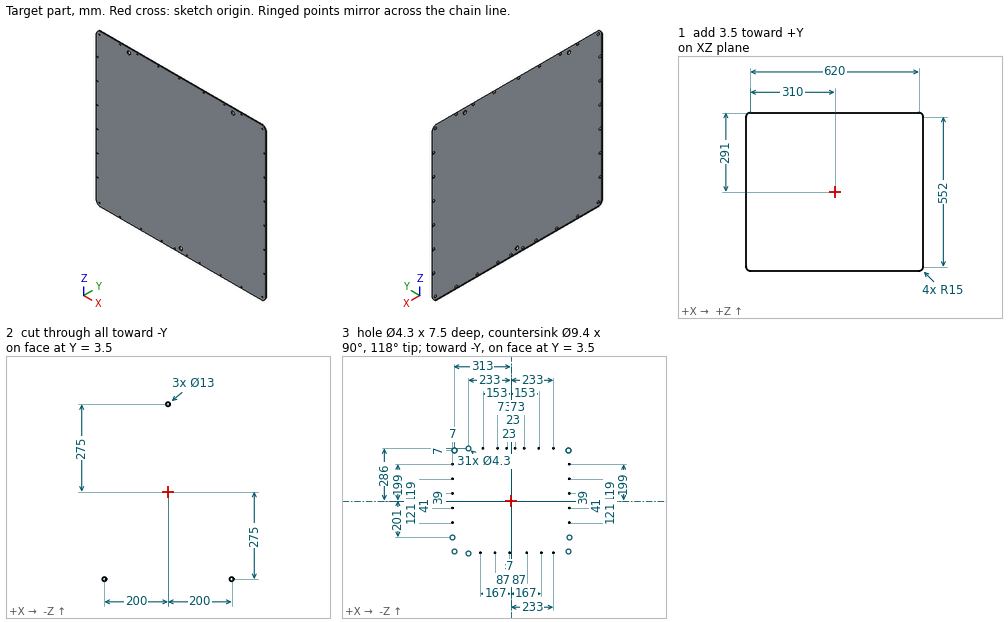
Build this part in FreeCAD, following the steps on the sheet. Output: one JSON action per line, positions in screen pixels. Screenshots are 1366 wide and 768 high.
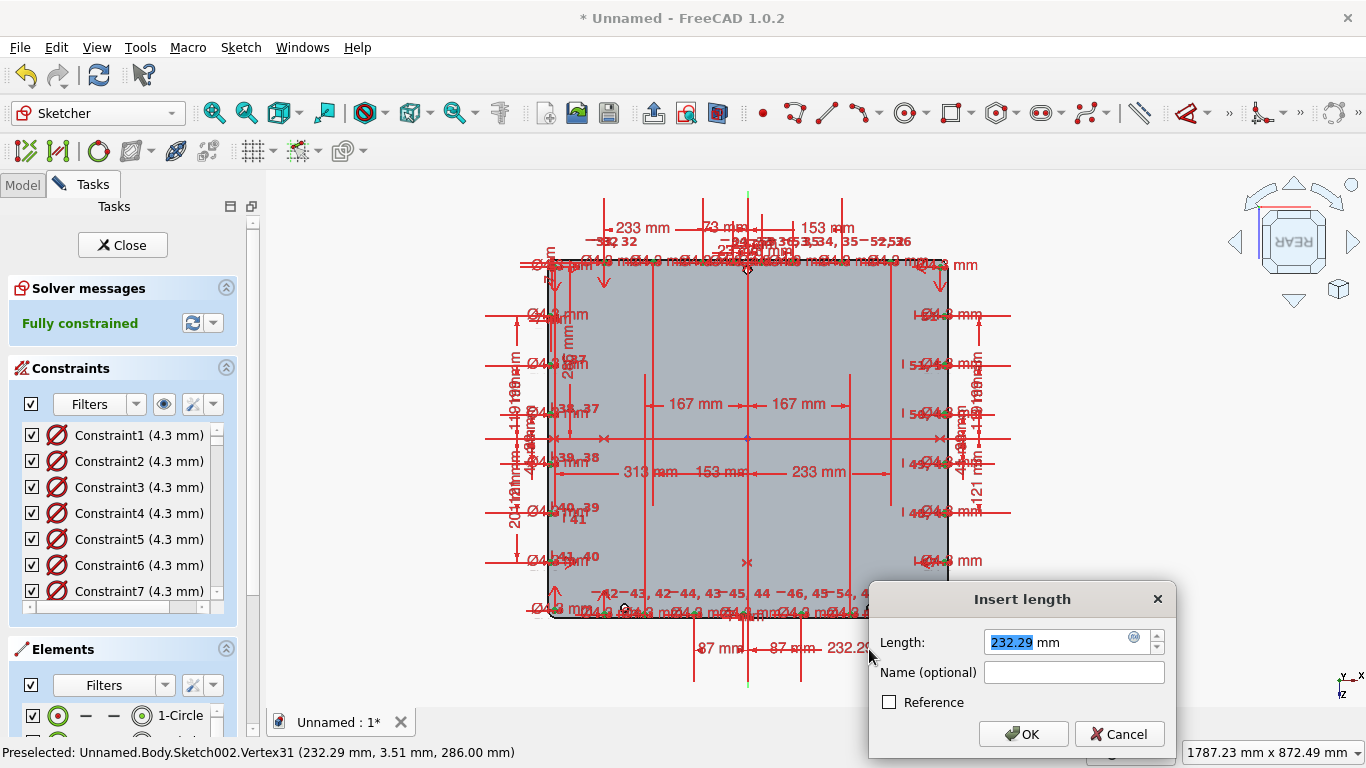
{"action": "type", "text": "233"}
{"action": "key", "text": "Return"}
{"action": "key", "text": "Escape"}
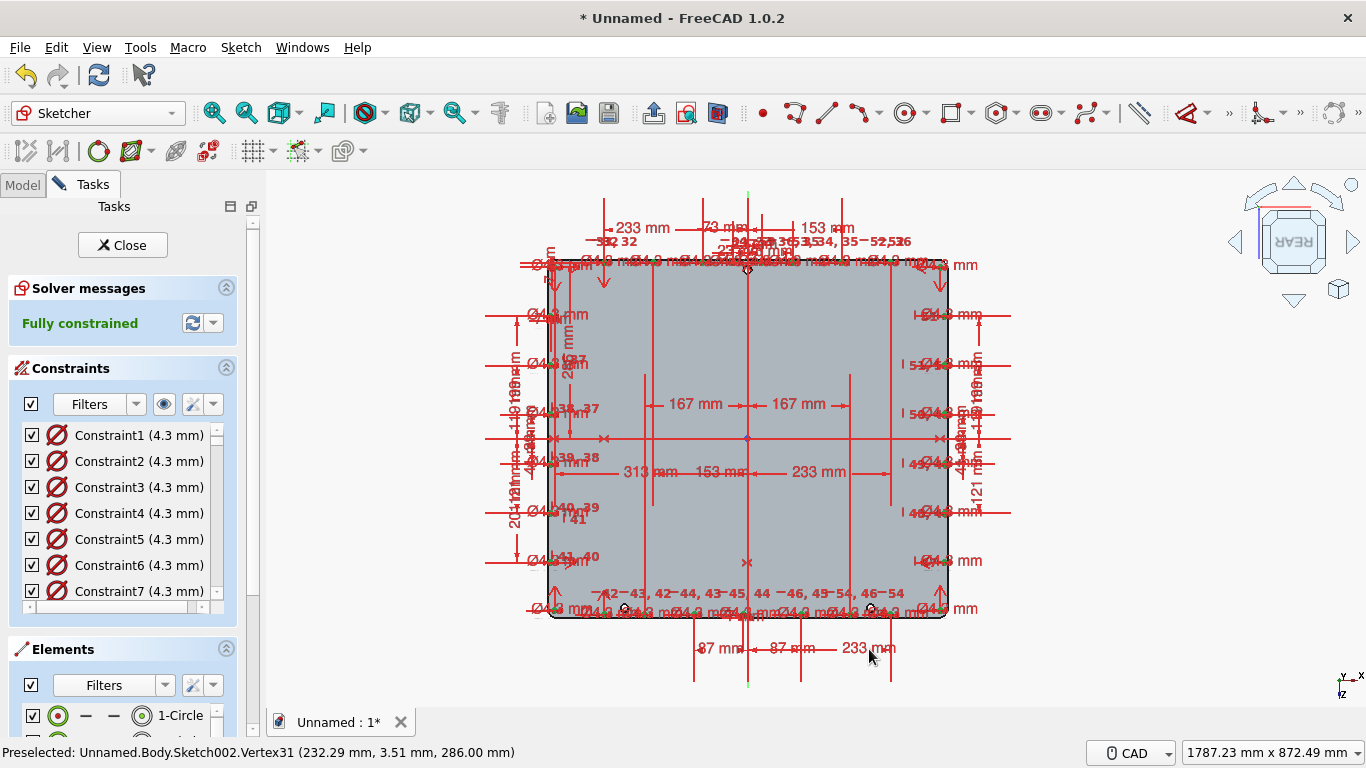
{"action": "left_click", "coordinate": [123, 245]}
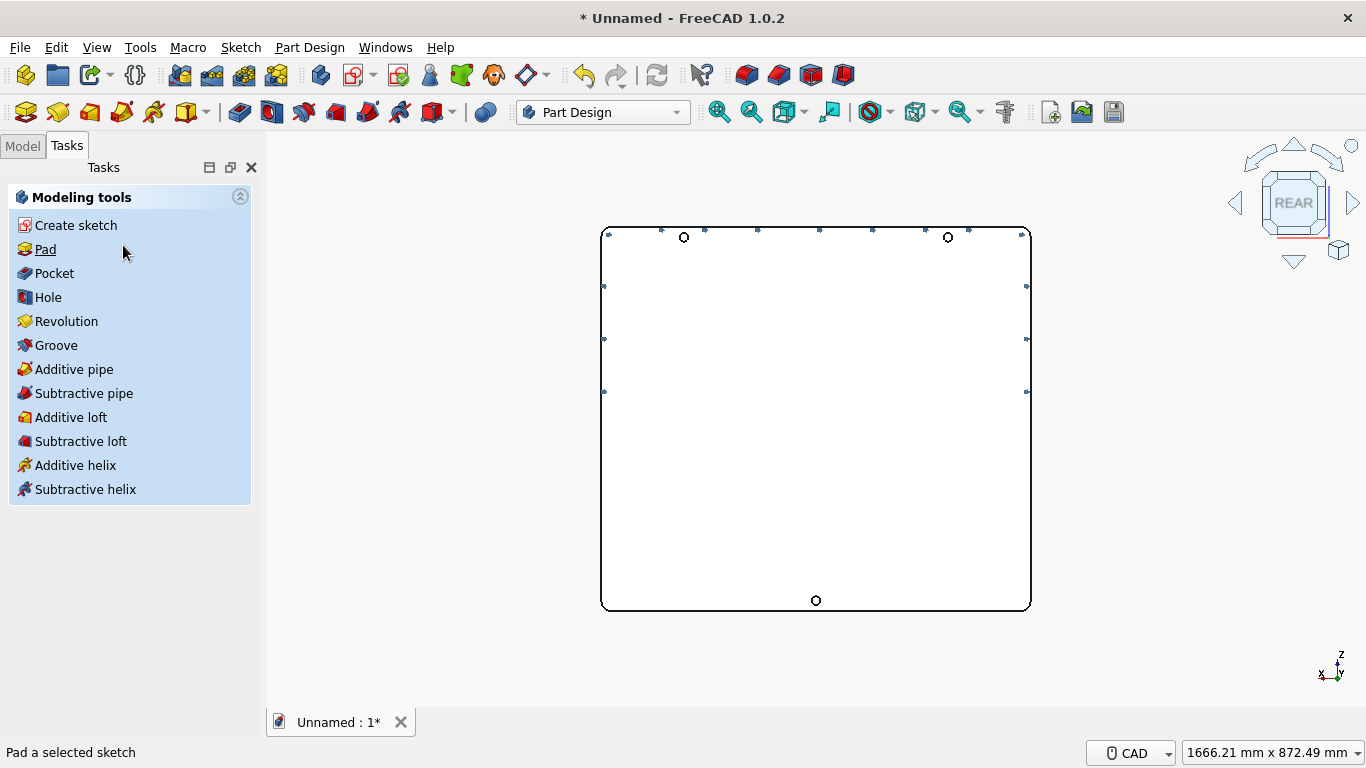
{"action": "left_click", "coordinate": [272, 112]}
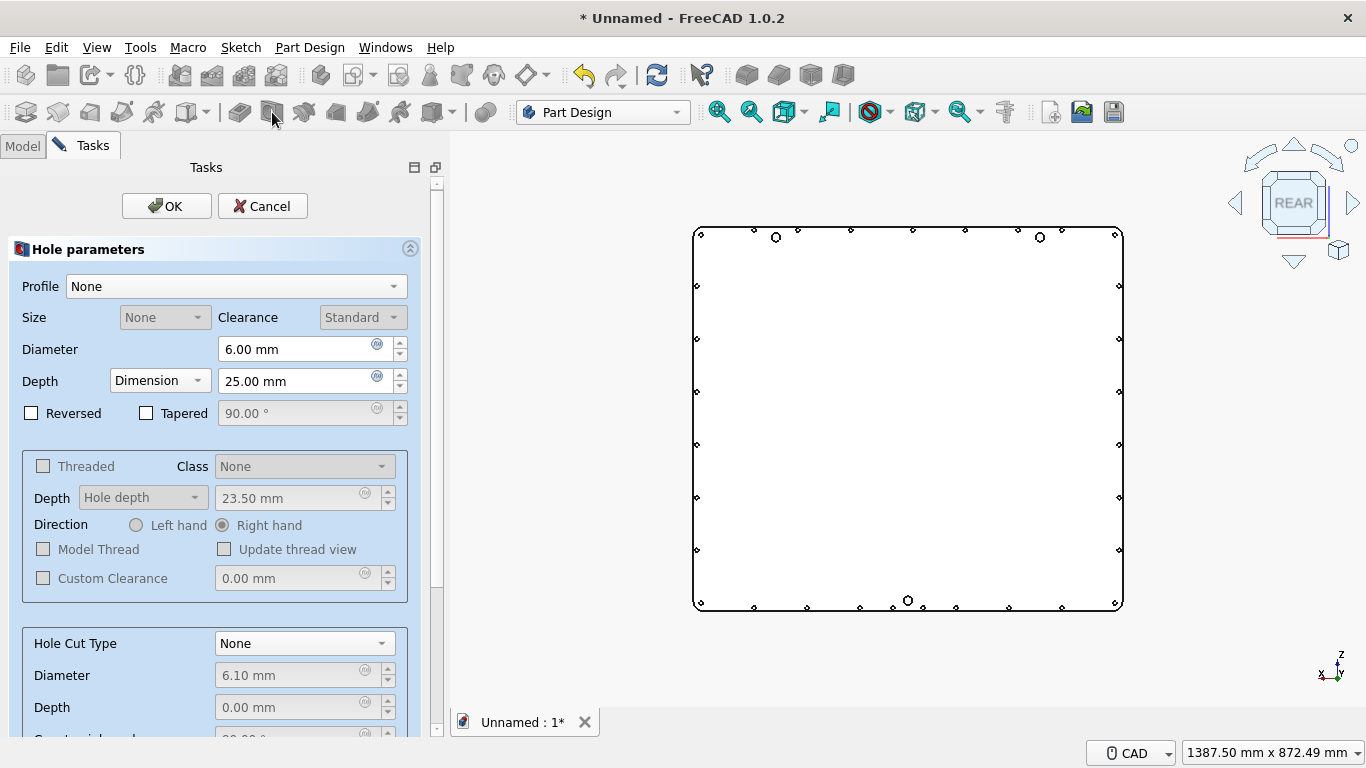
{"action": "triple_click", "coordinate": [305, 349]}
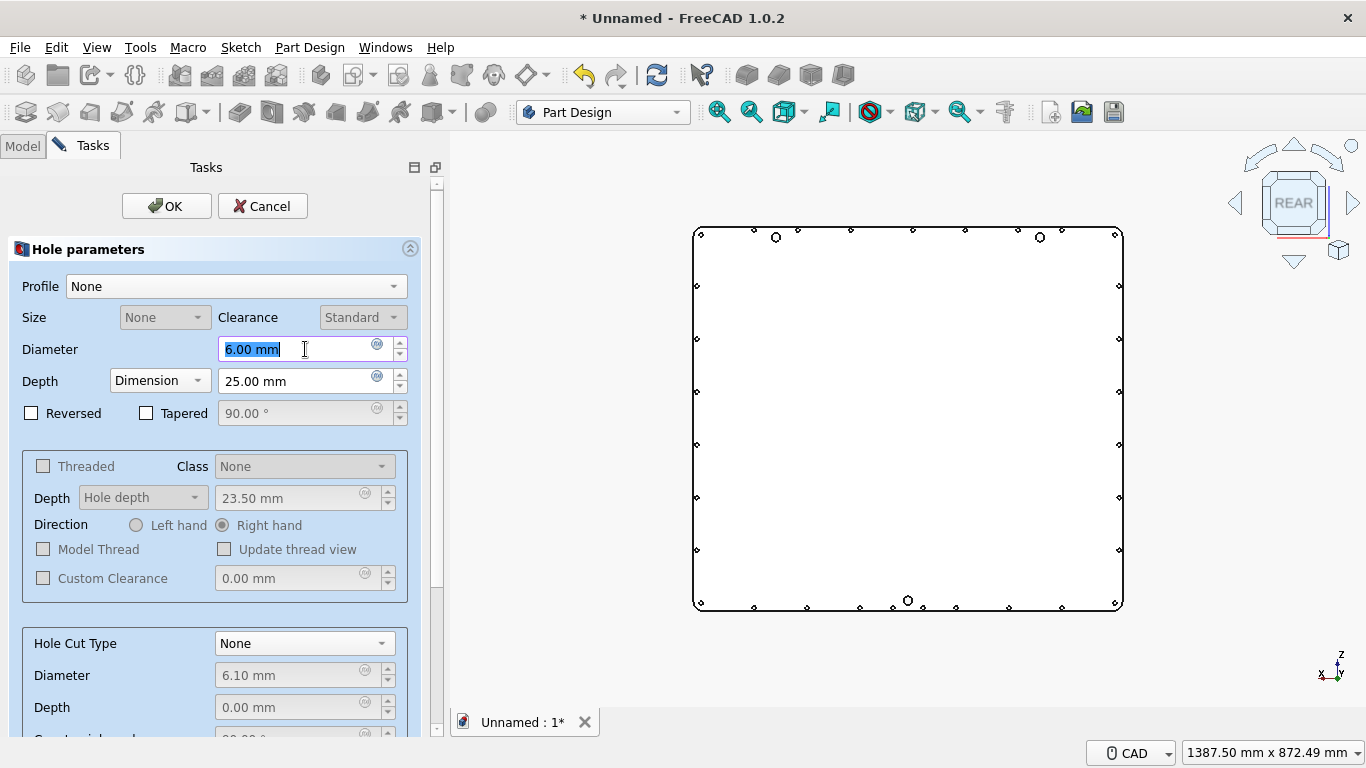
{"action": "type", "text": "4.3"}
{"action": "key", "text": "Tab"}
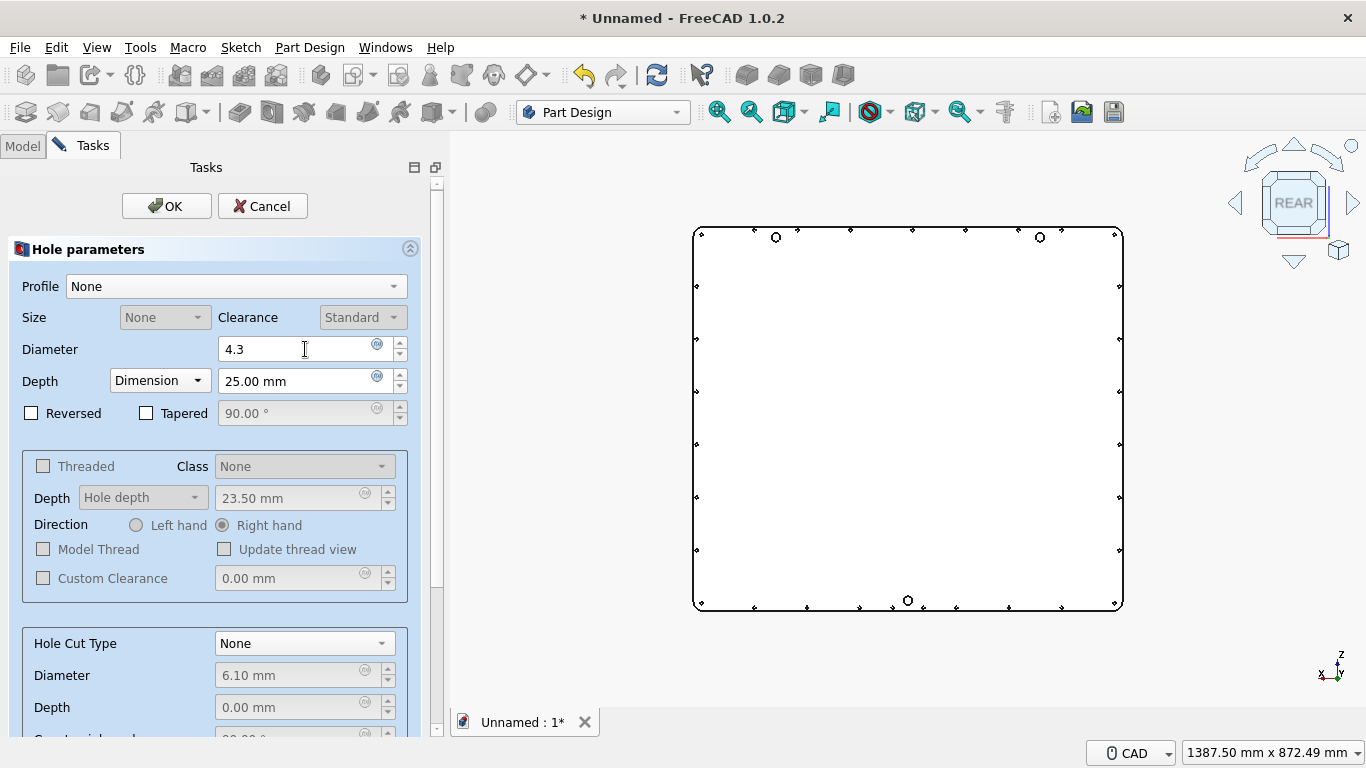
{"action": "triple_click", "coordinate": [305, 381]}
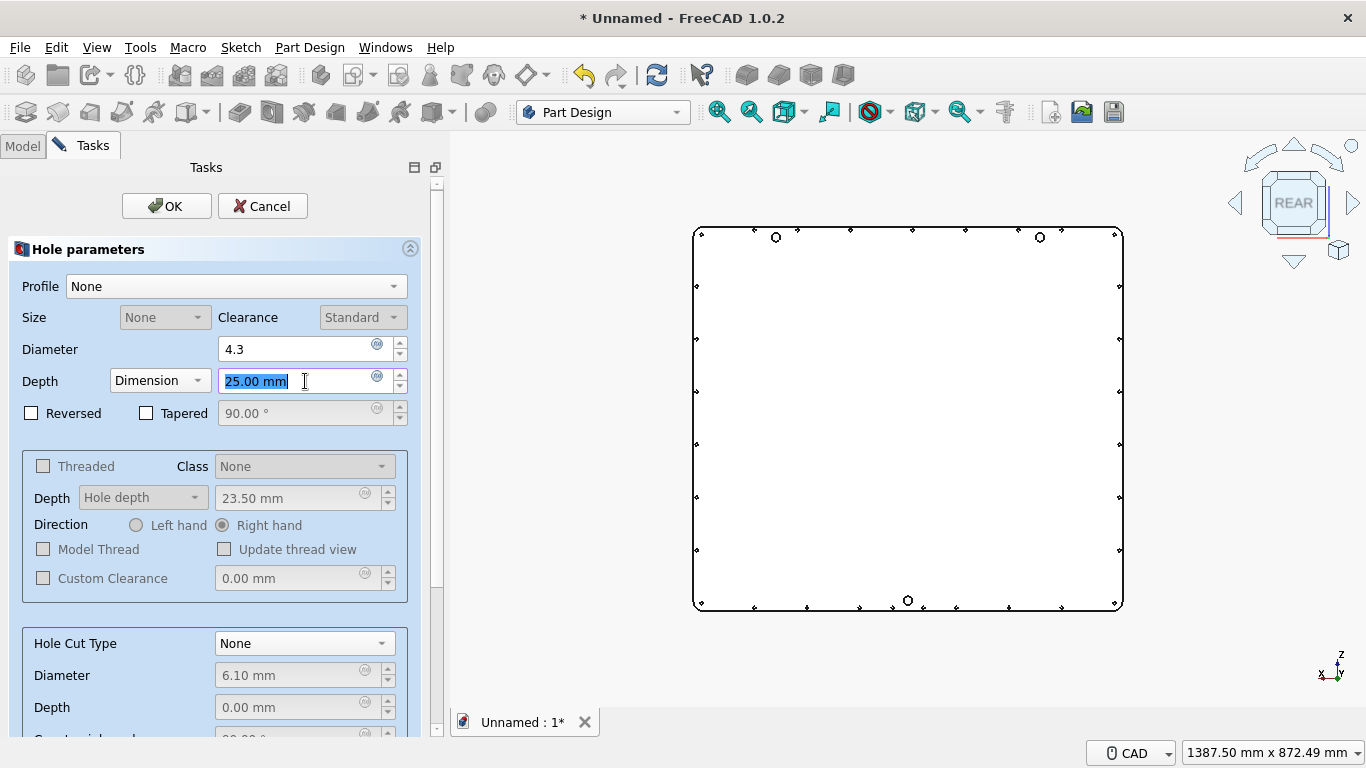
{"action": "type", "text": "7.5"}
{"action": "key", "text": "Tab"}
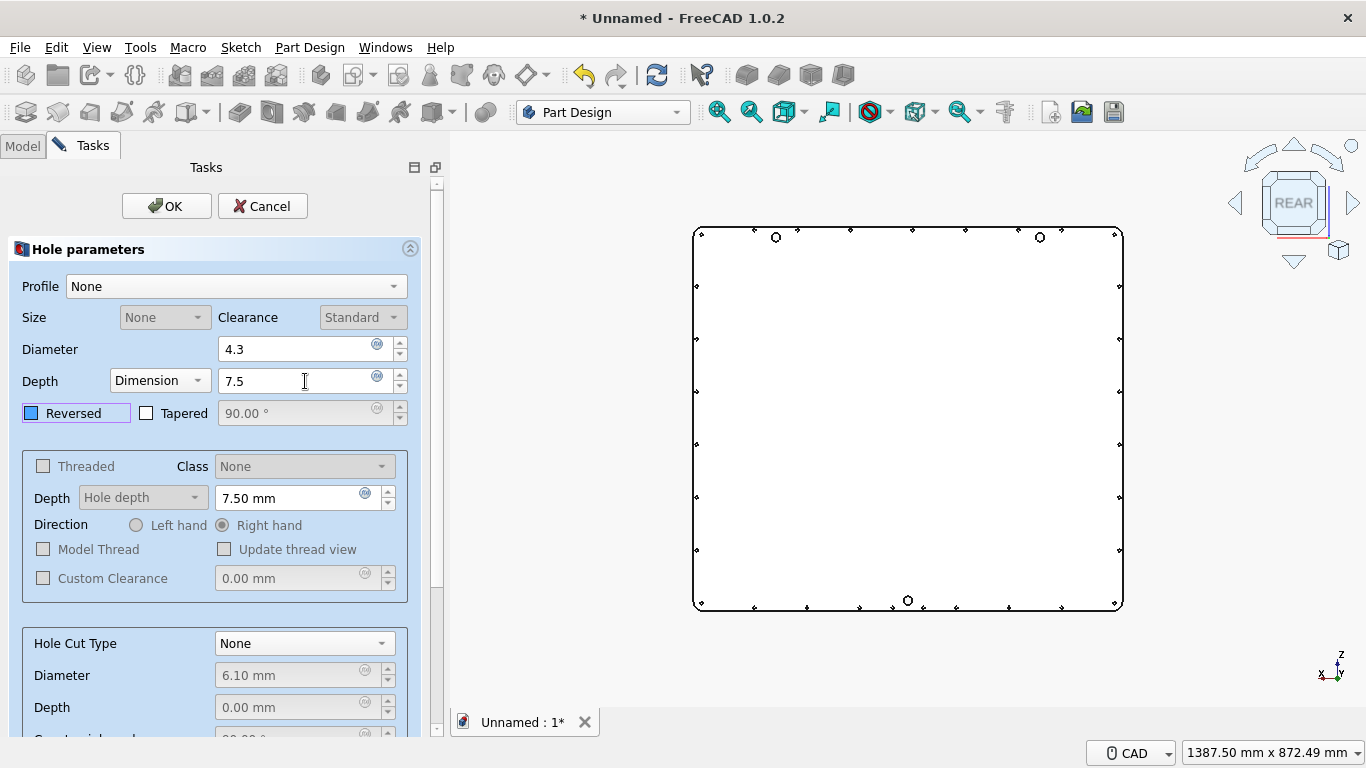
{"action": "left_click", "coordinate": [306, 644]}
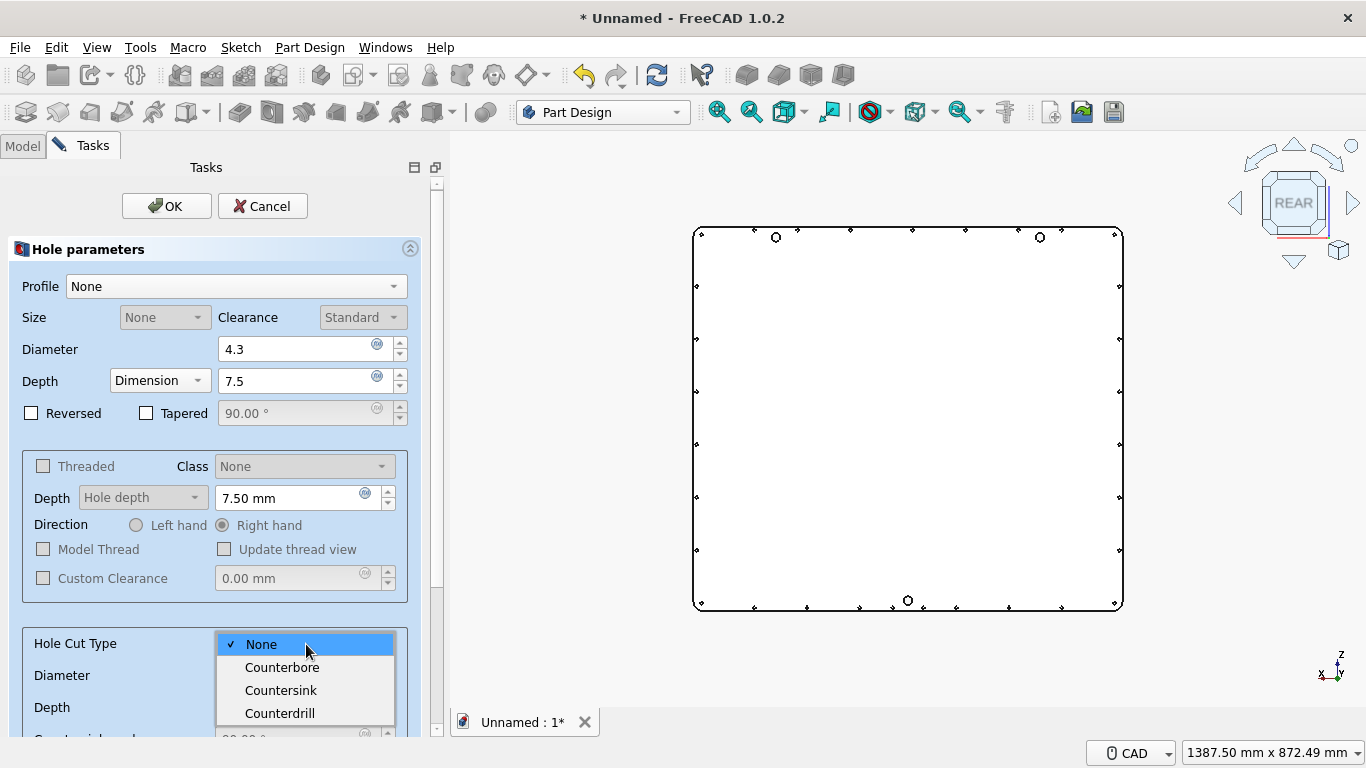
{"action": "left_click", "coordinate": [304, 690]}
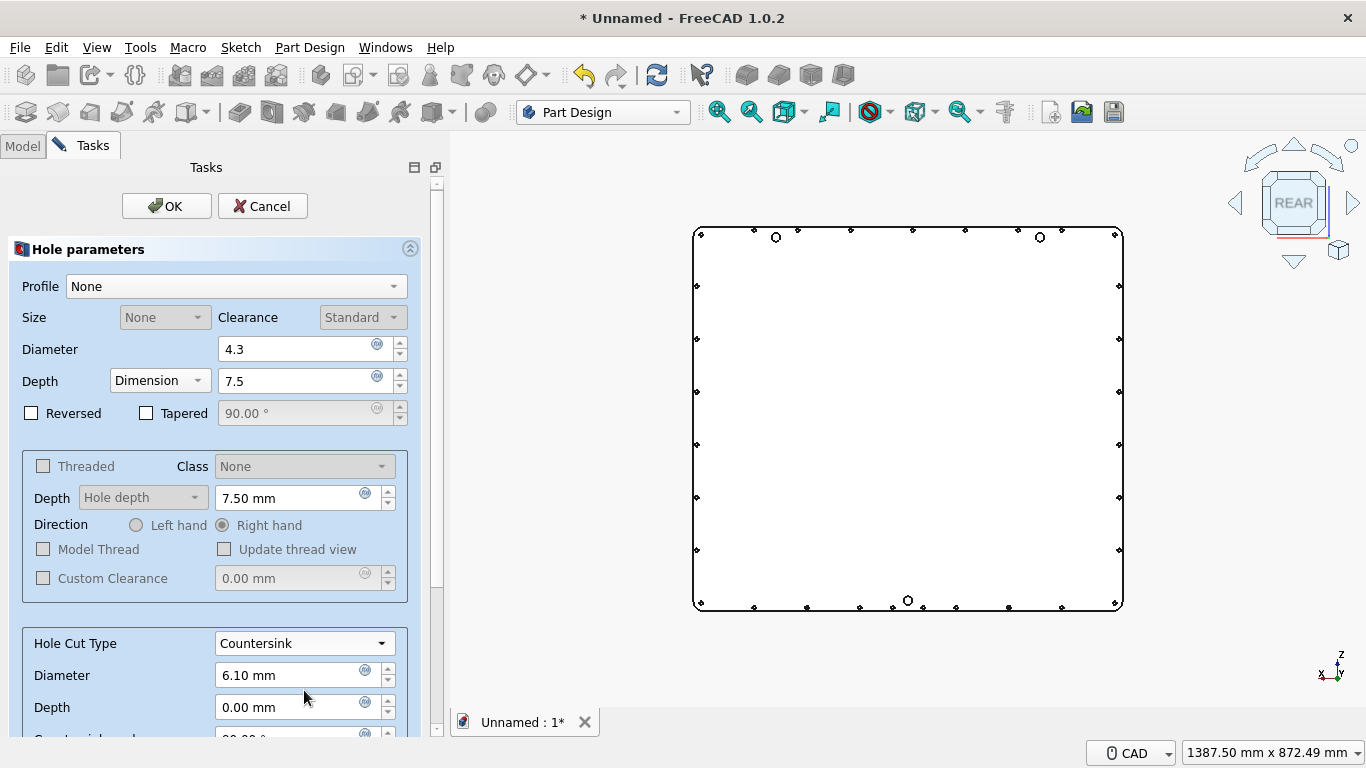
{"action": "triple_click", "coordinate": [298, 675]}